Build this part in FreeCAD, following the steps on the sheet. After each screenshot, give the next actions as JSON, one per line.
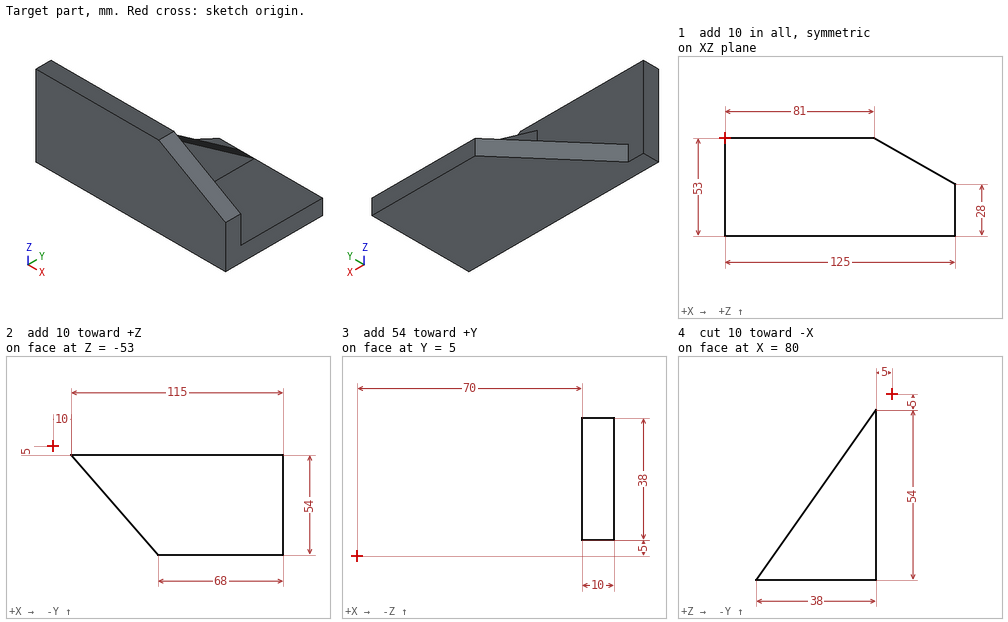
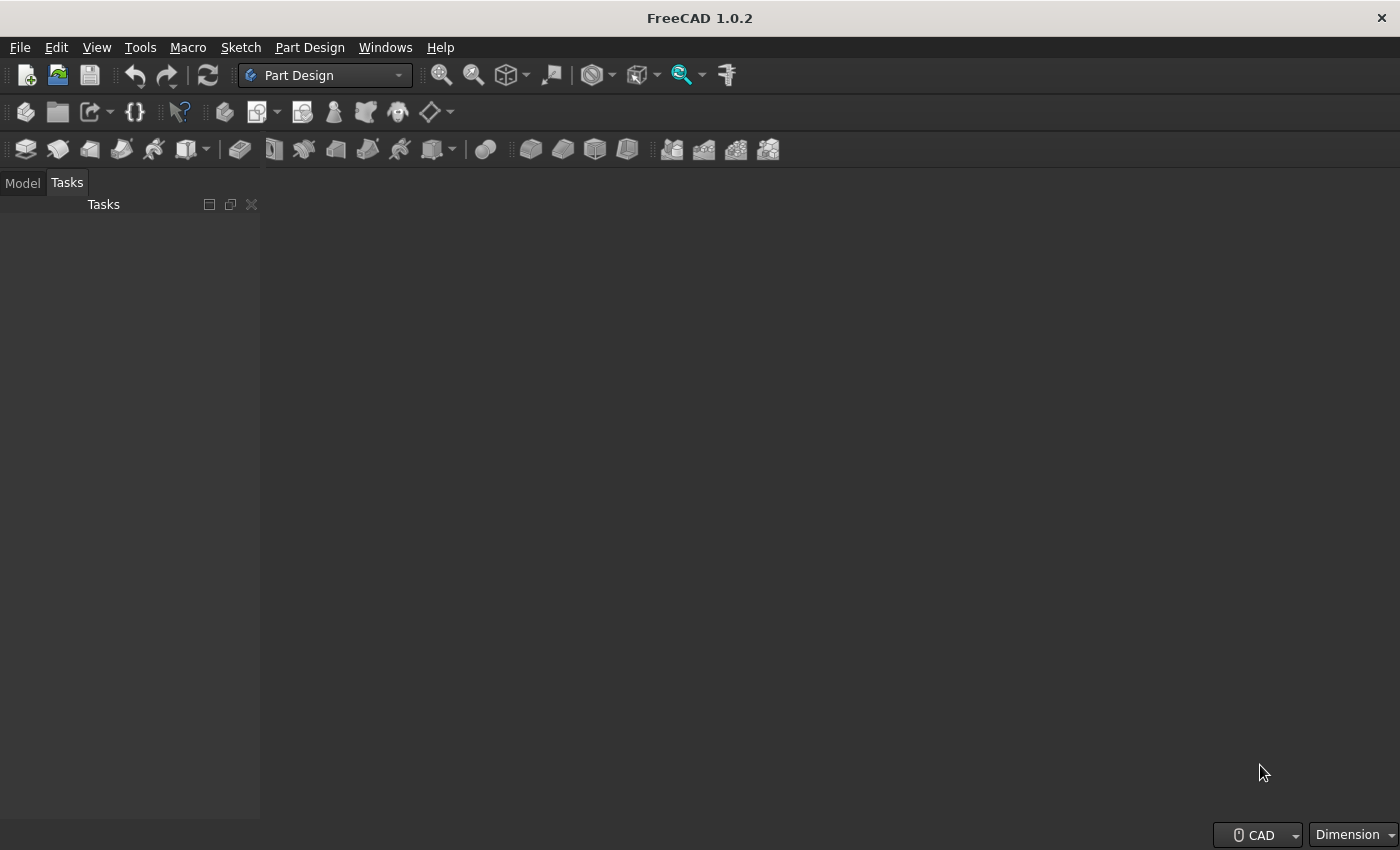
{"action": "left_click", "coordinate": [26, 76]}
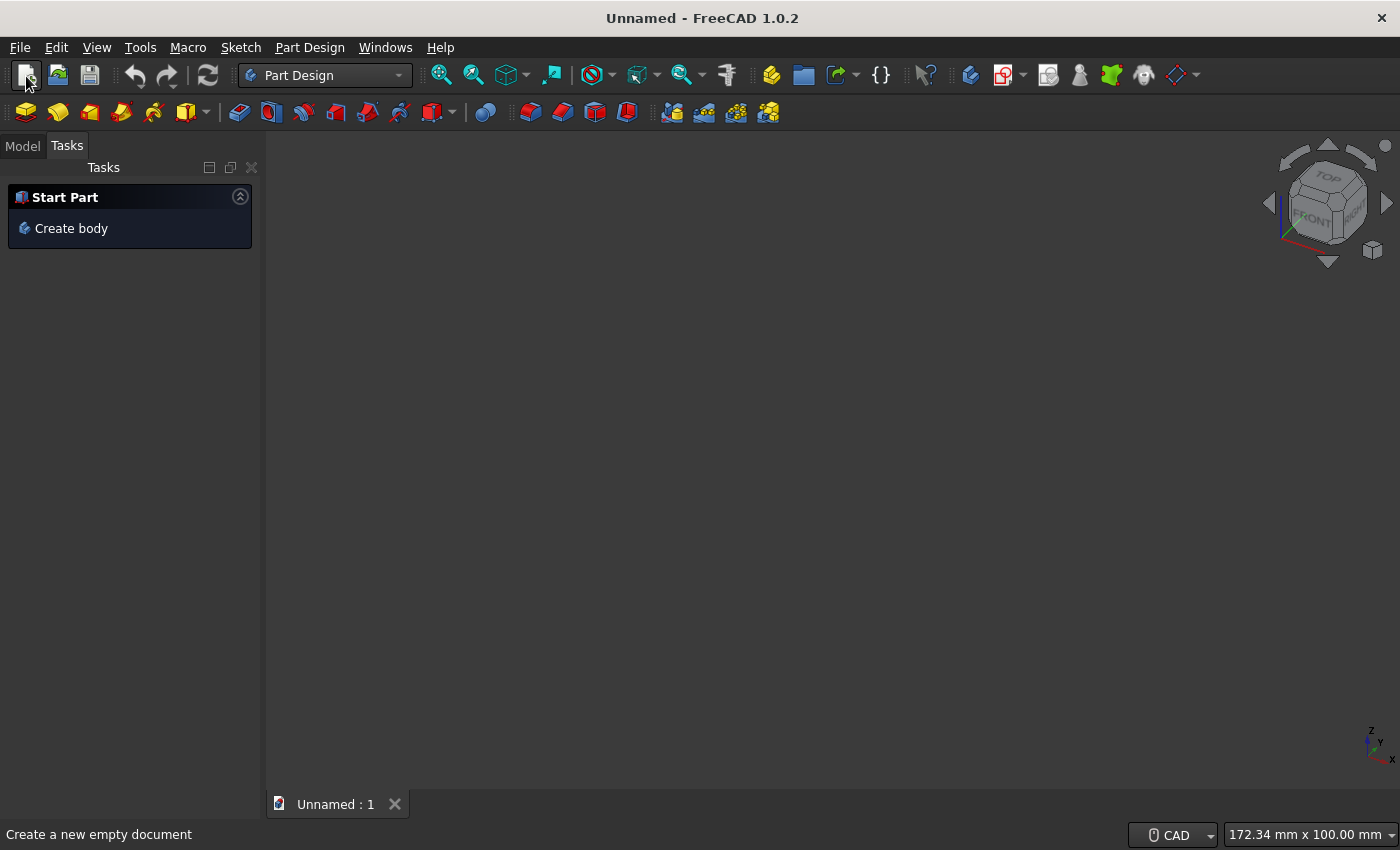
{"action": "left_click", "coordinate": [1004, 76]}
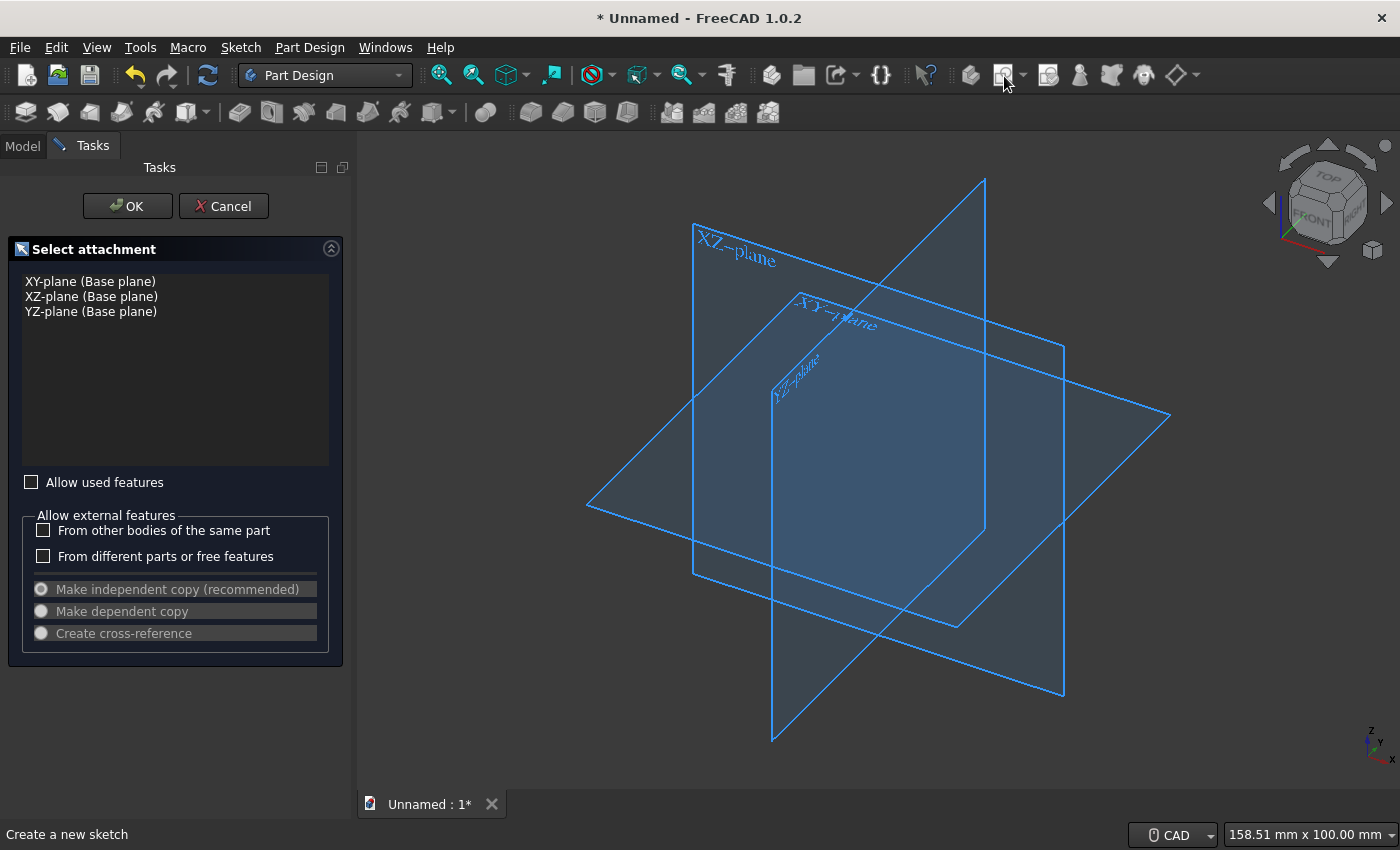
{"action": "left_click", "coordinate": [82, 296]}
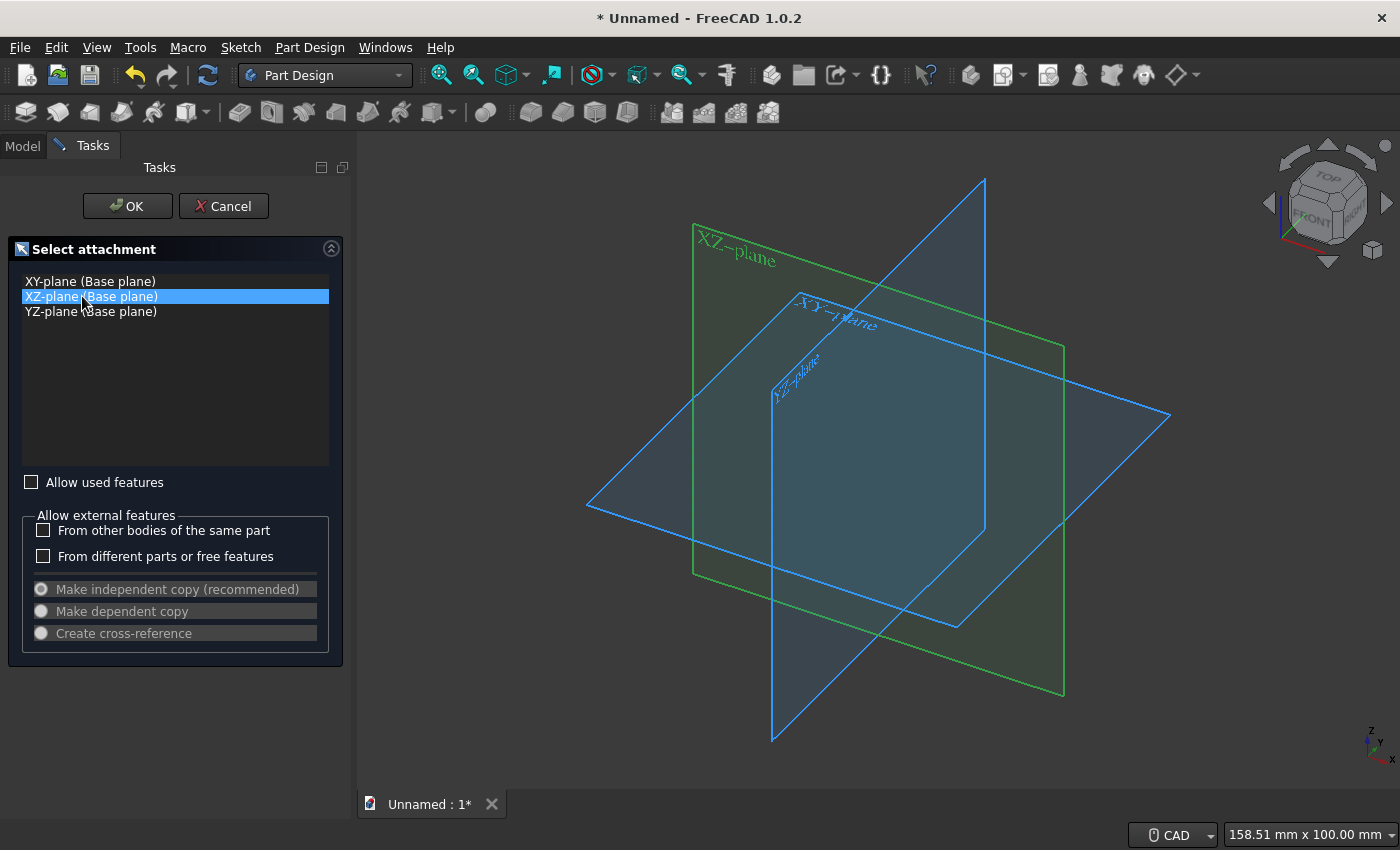
{"action": "left_click", "coordinate": [128, 206]}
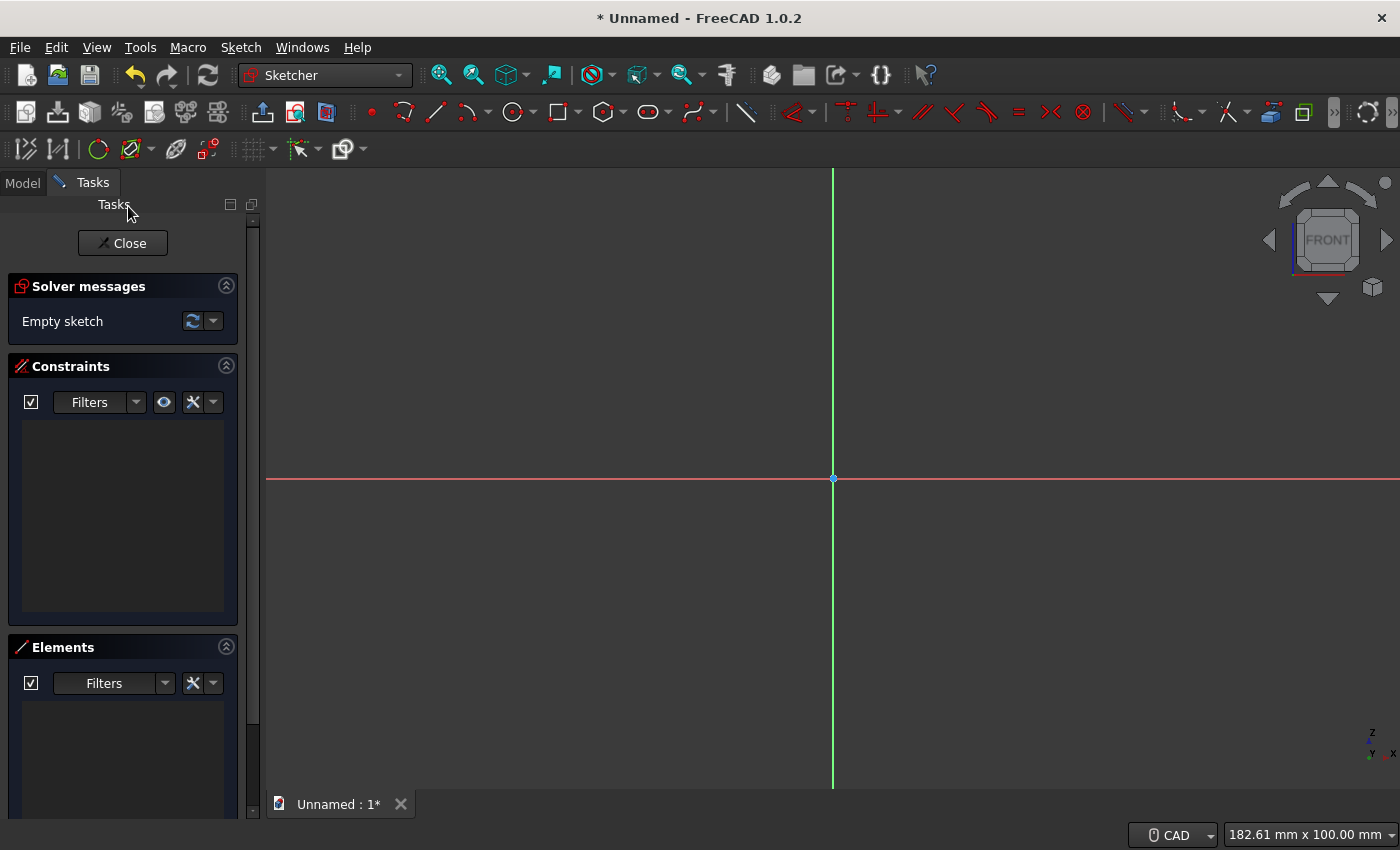
{"action": "scroll", "coordinate": [294, 196], "scroll_direction": "down", "scroll_amount": 2}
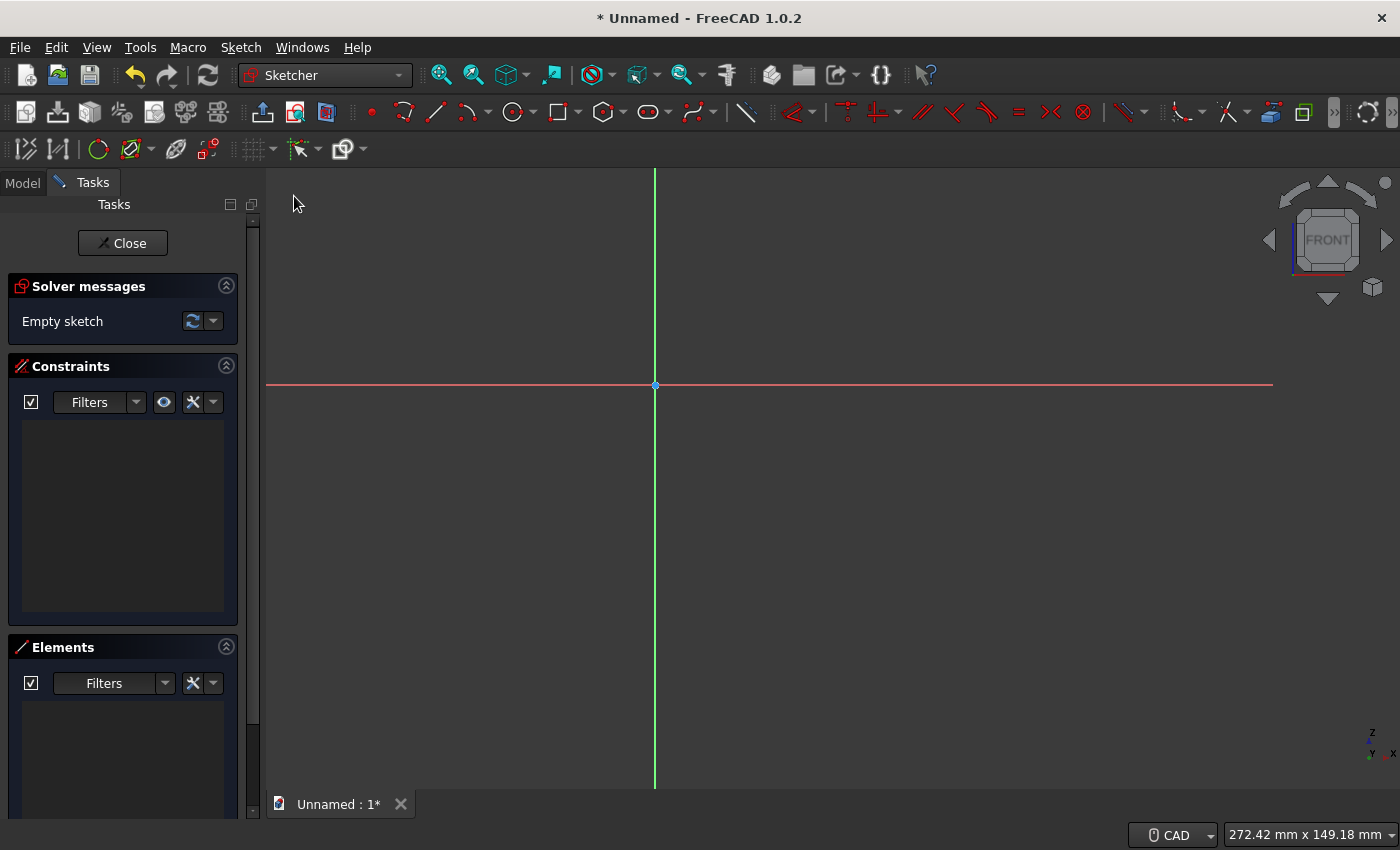
{"action": "key", "text": "g m"}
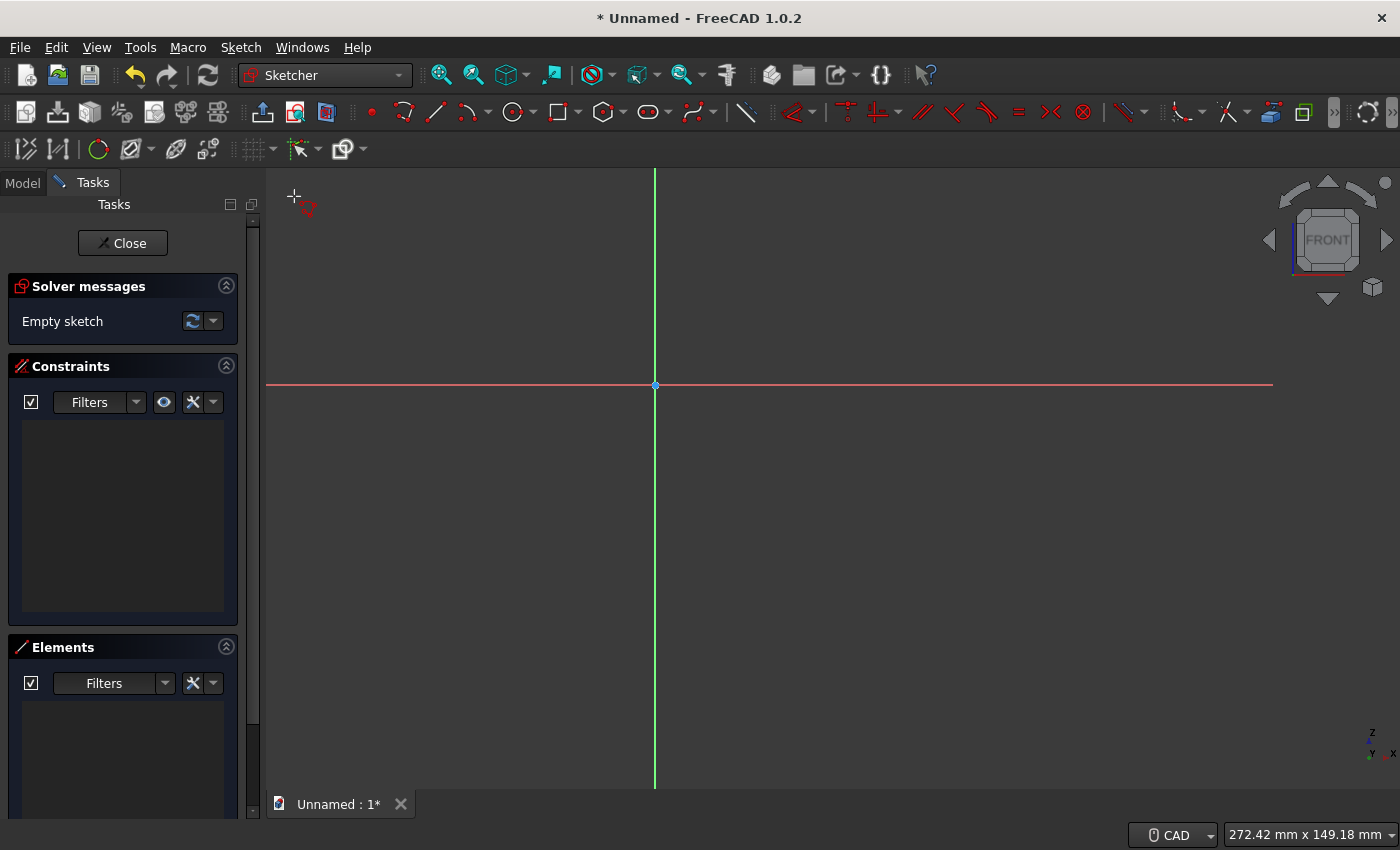
{"action": "left_click", "coordinate": [655, 385]}
{"action": "left_click", "coordinate": [992, 394]}
{"action": "left_click", "coordinate": [1176, 489]}
{"action": "left_click", "coordinate": [1176, 606]}
{"action": "left_click", "coordinate": [664, 606]}
{"action": "left_click", "coordinate": [655, 385]}
{"action": "key", "text": "Escape"}
{"action": "key", "text": "Escape"}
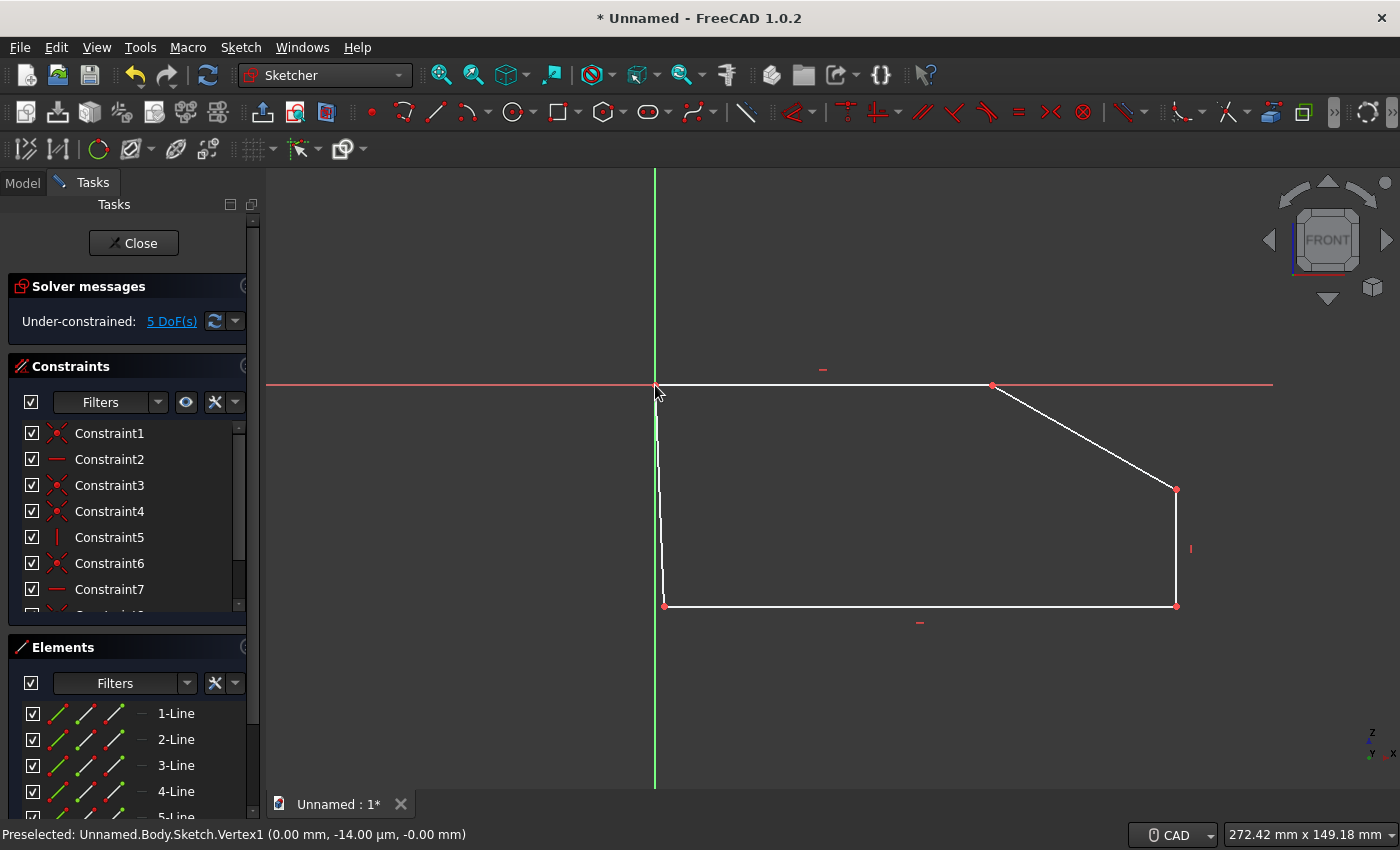
{"action": "left_click", "coordinate": [658, 452]}